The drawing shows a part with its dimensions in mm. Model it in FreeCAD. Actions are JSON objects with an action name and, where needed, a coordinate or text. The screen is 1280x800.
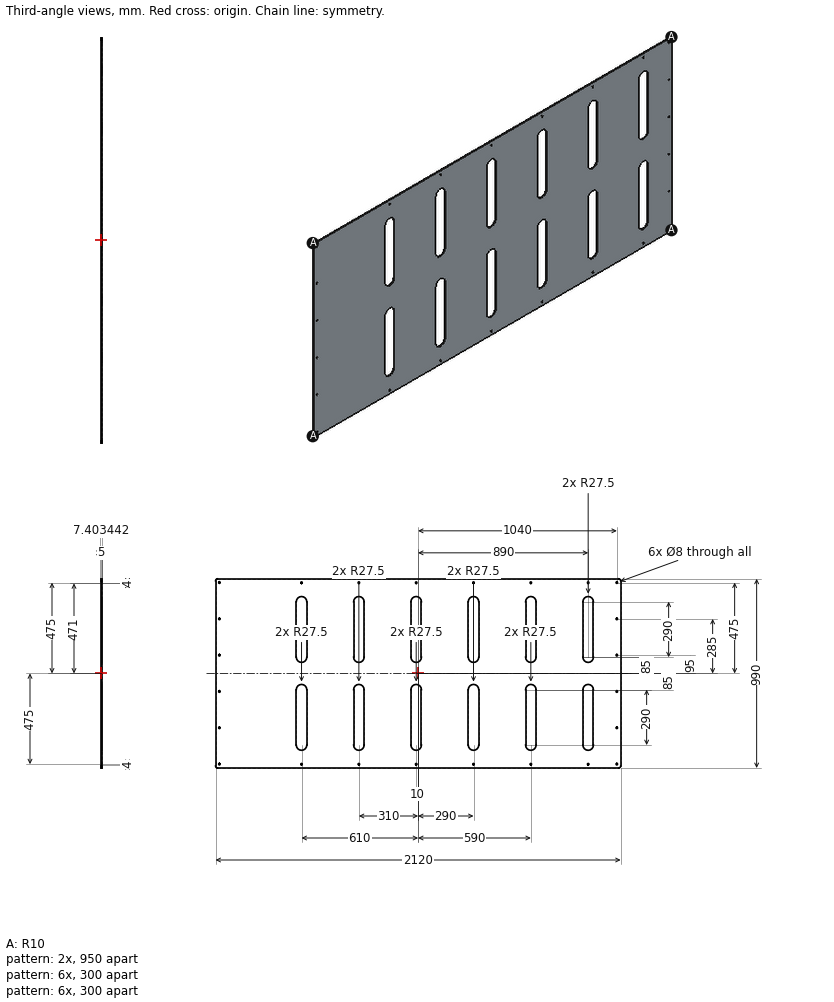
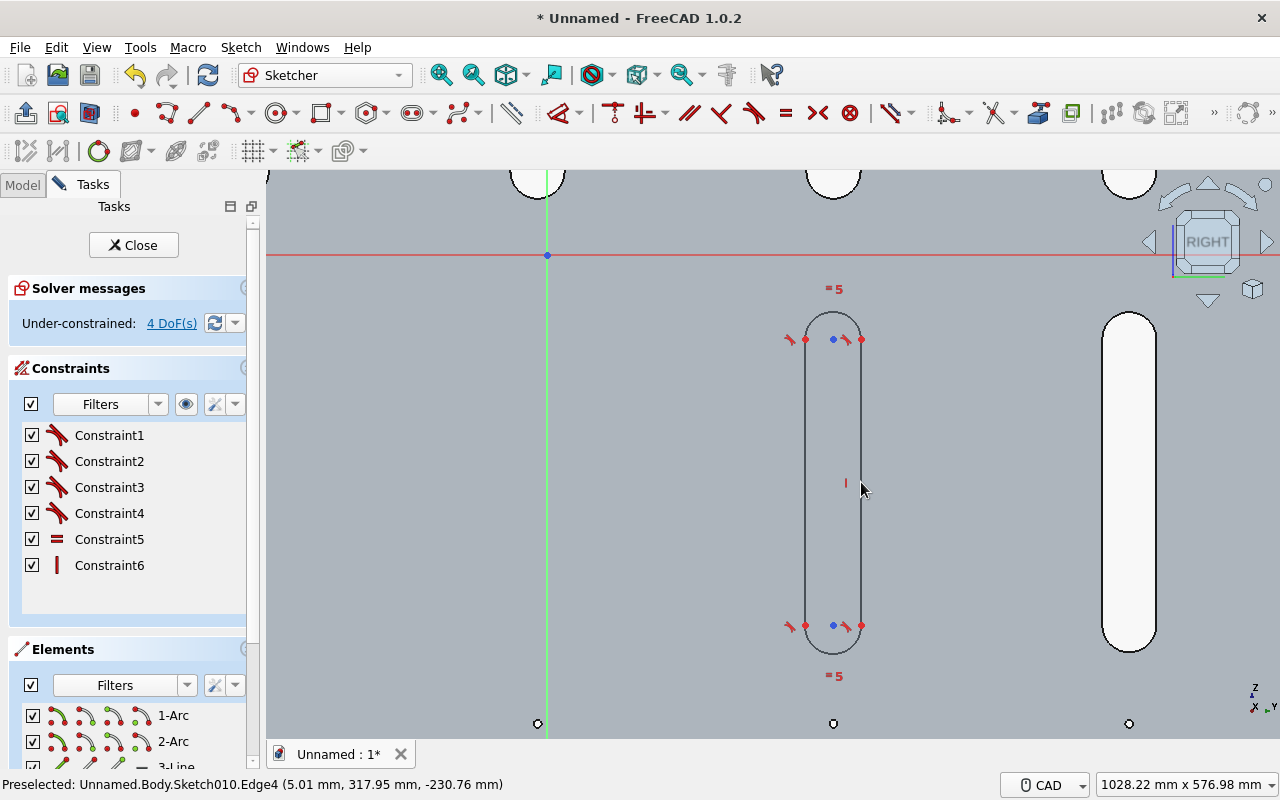
{"action": "left_click", "coordinate": [558, 114]}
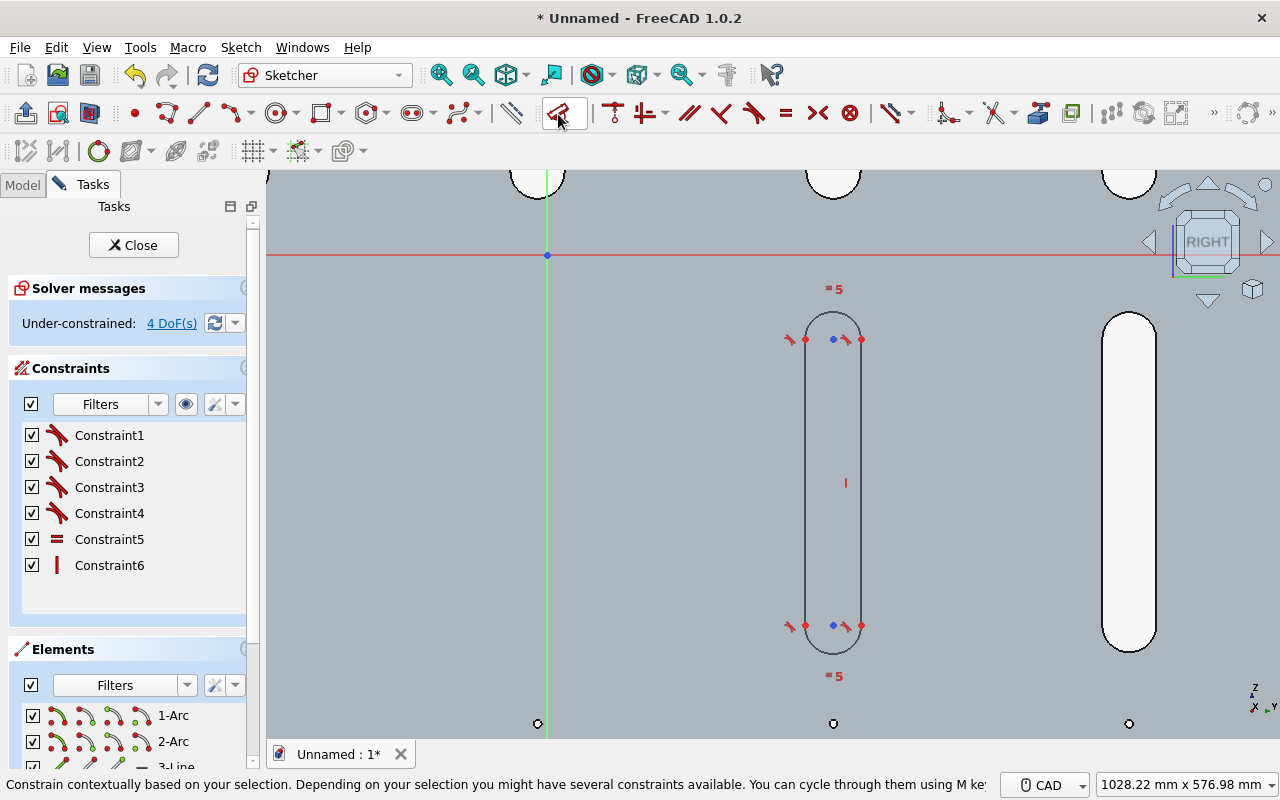
{"action": "scroll", "coordinate": [817, 649], "scroll_direction": "up", "scroll_amount": 2}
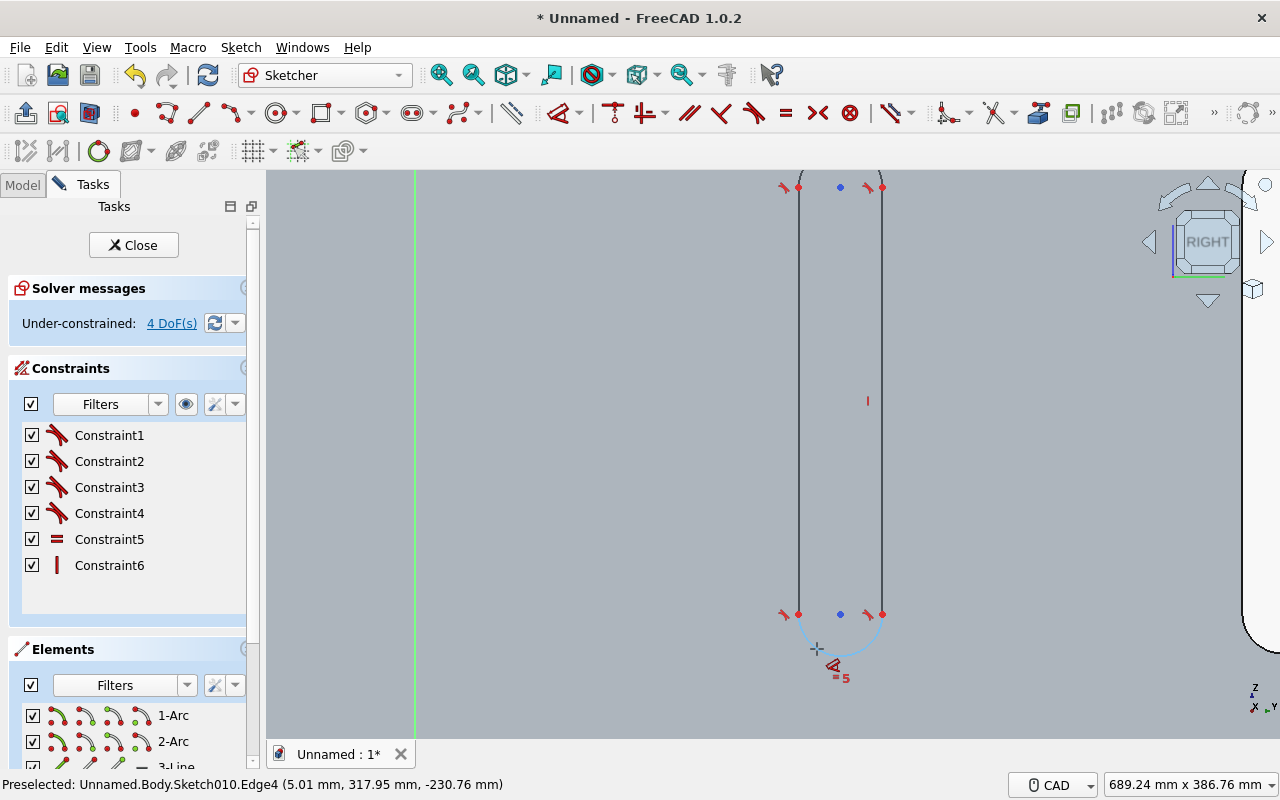
{"action": "left_click", "coordinate": [816, 648]}
{"action": "left_click", "coordinate": [797, 674]}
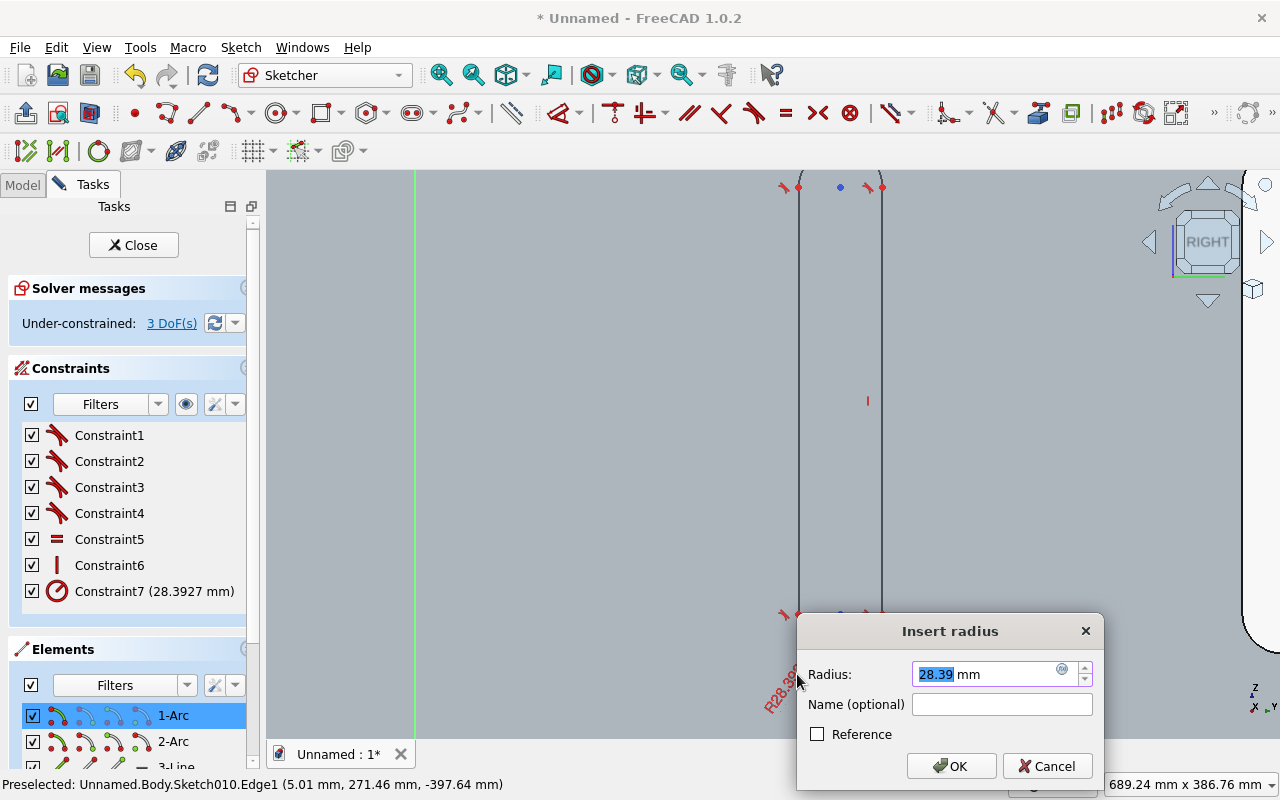
{"action": "type", "text": "27.5"}
{"action": "key", "text": "Return"}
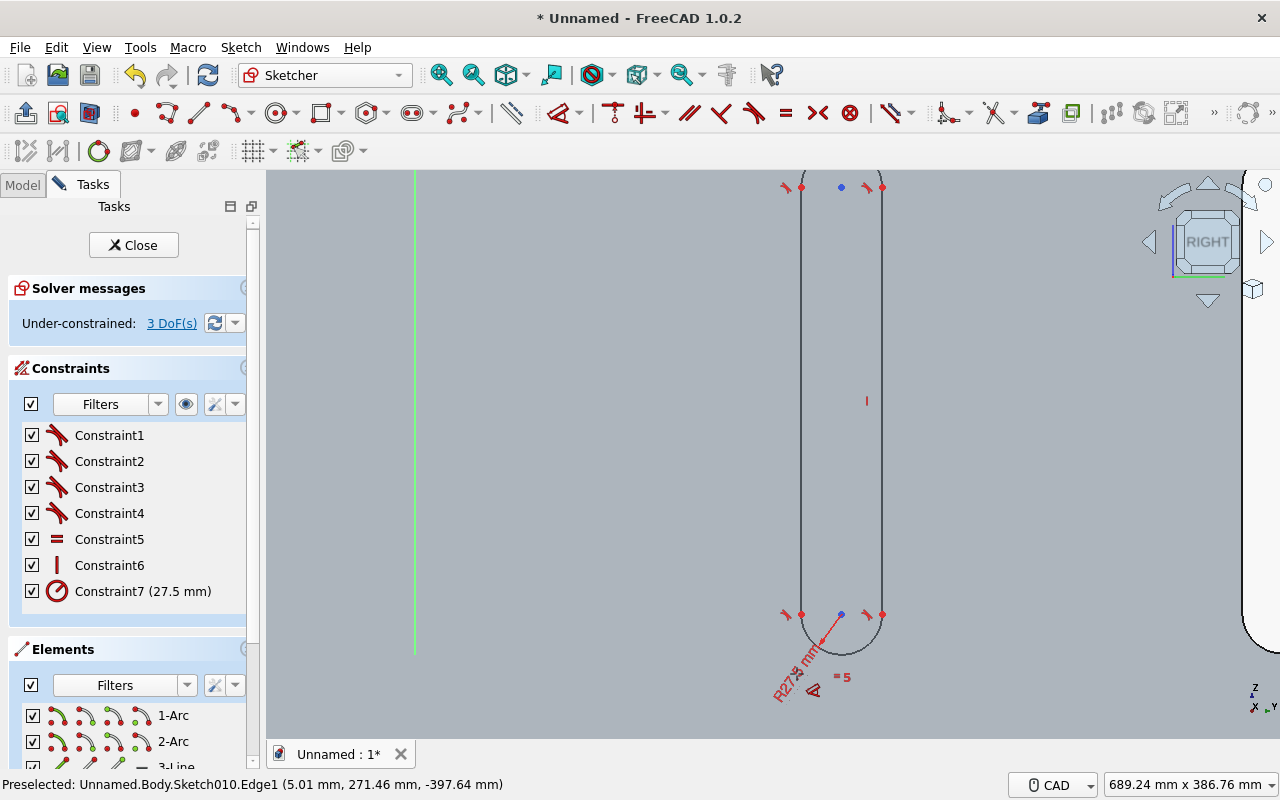
{"action": "left_click", "coordinate": [801, 486]}
{"action": "left_click", "coordinate": [835, 406]}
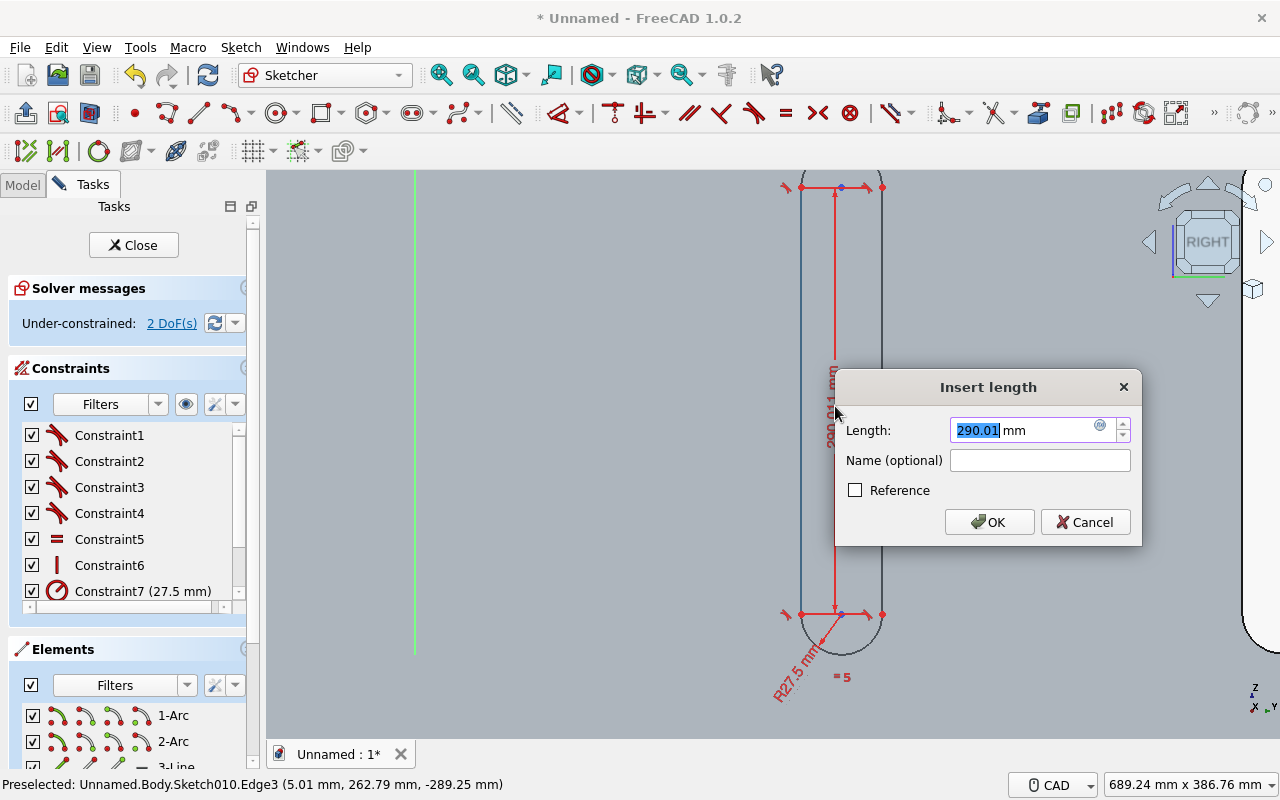
{"action": "type", "text": "290"}
{"action": "key", "text": "Return"}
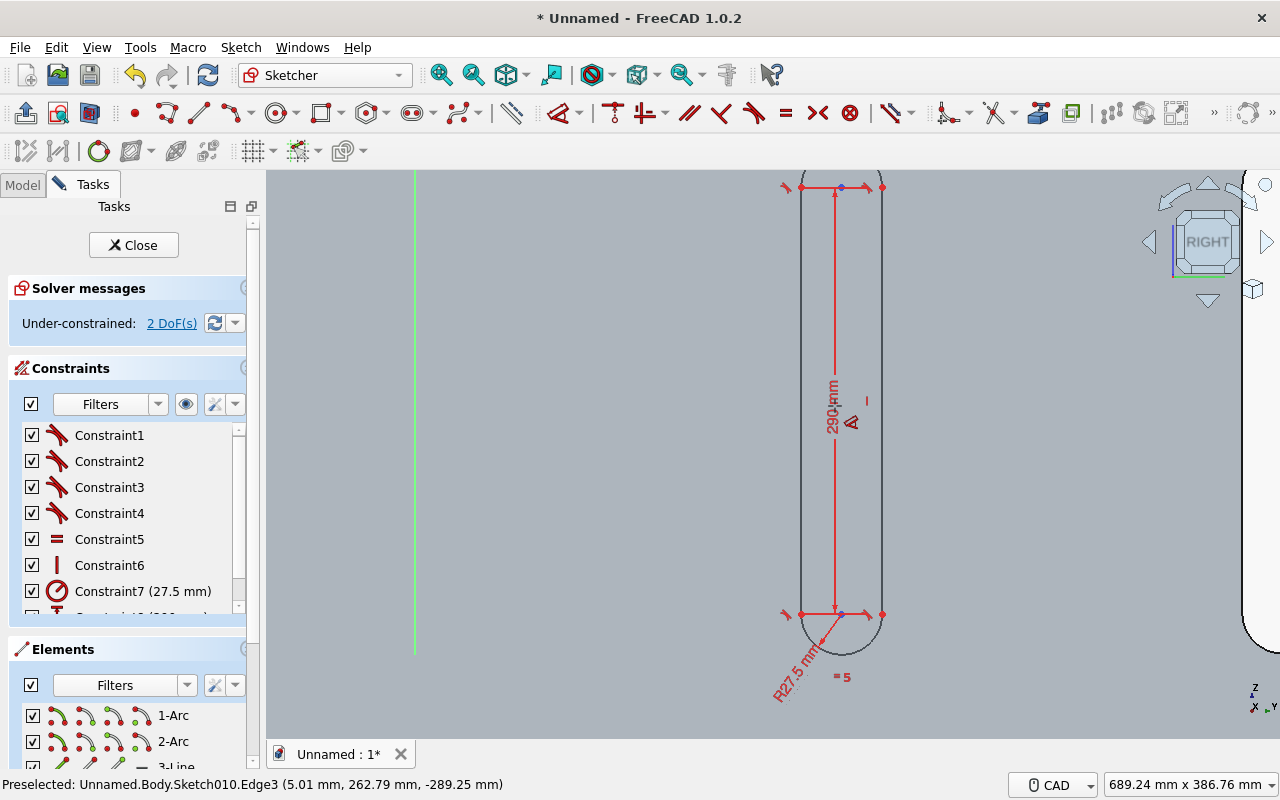
{"action": "scroll", "coordinate": [819, 652], "scroll_direction": "down", "scroll_amount": 2}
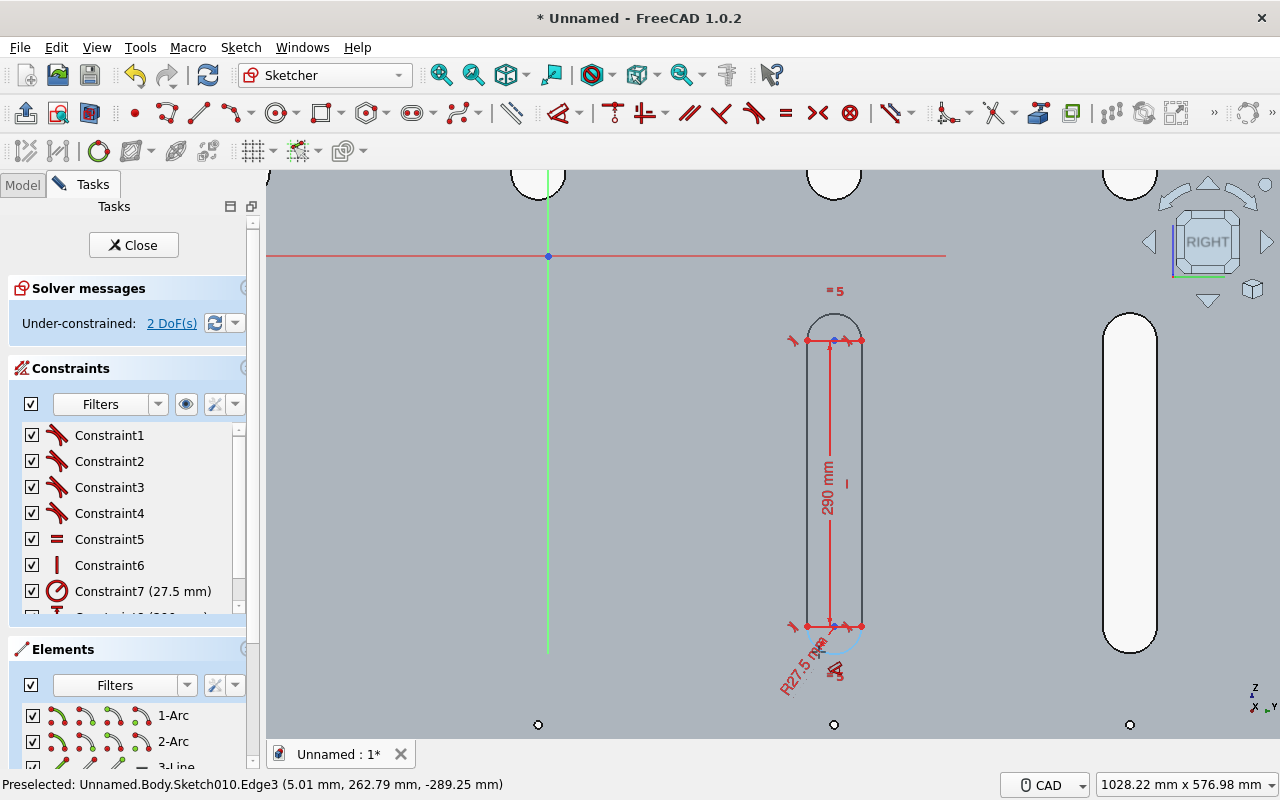
{"action": "left_click", "coordinate": [862, 341]}
{"action": "left_click", "coordinate": [896, 299]}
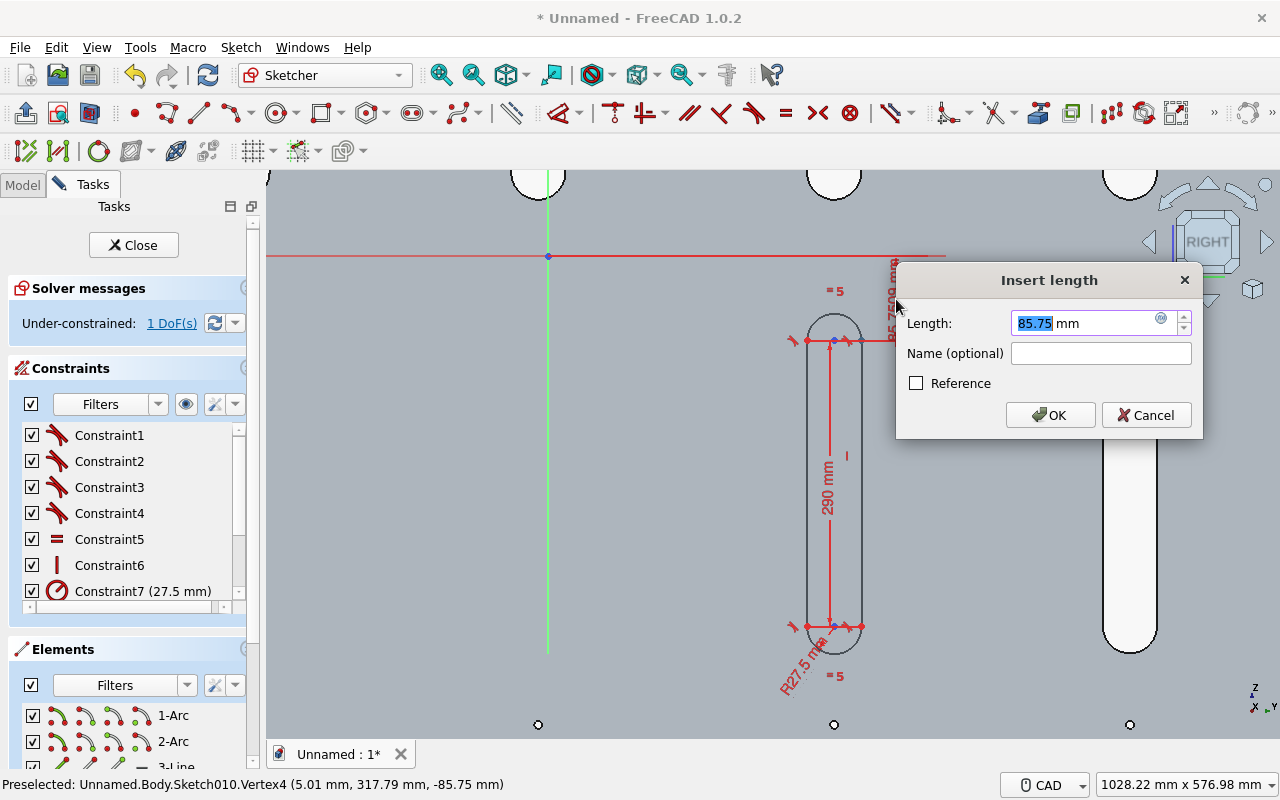
{"action": "type", "text": "85"}
{"action": "key", "text": "Return"}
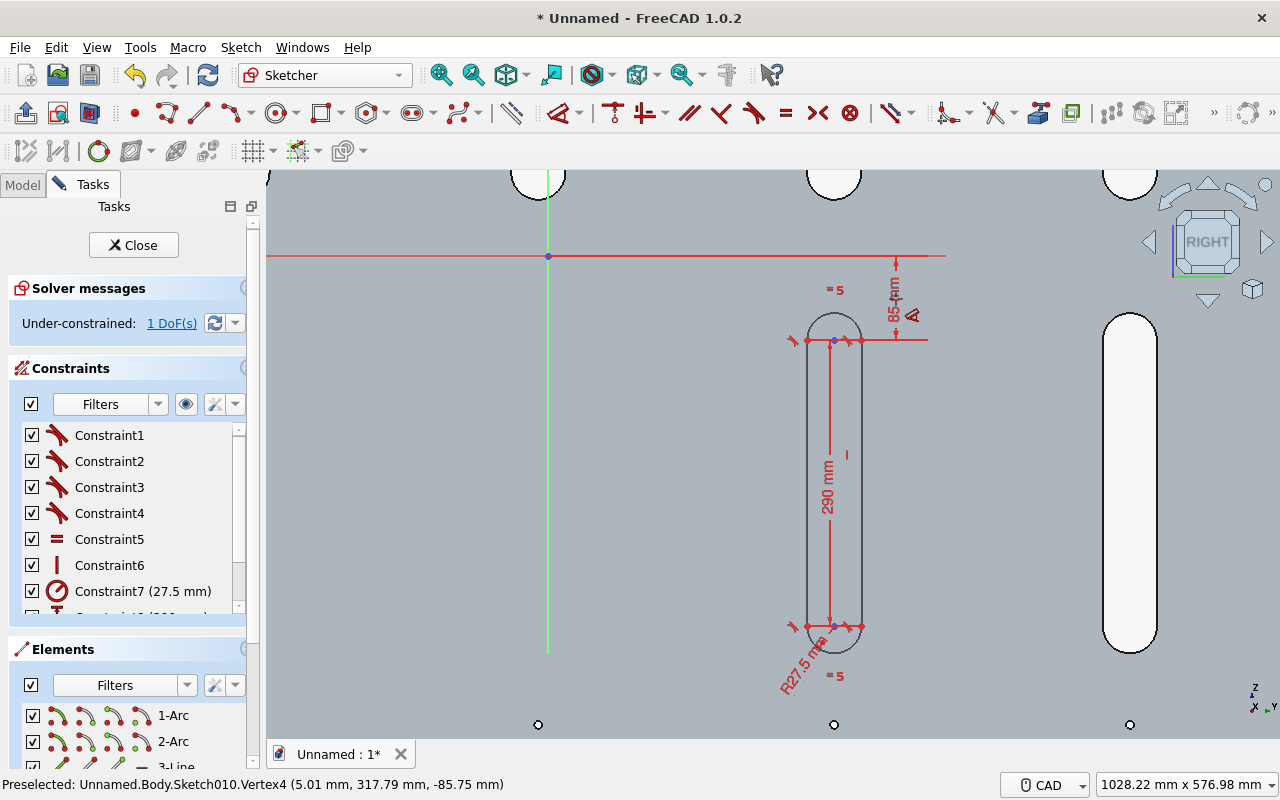
{"action": "left_click", "coordinate": [834, 626]}
{"action": "left_click", "coordinate": [691, 222]}